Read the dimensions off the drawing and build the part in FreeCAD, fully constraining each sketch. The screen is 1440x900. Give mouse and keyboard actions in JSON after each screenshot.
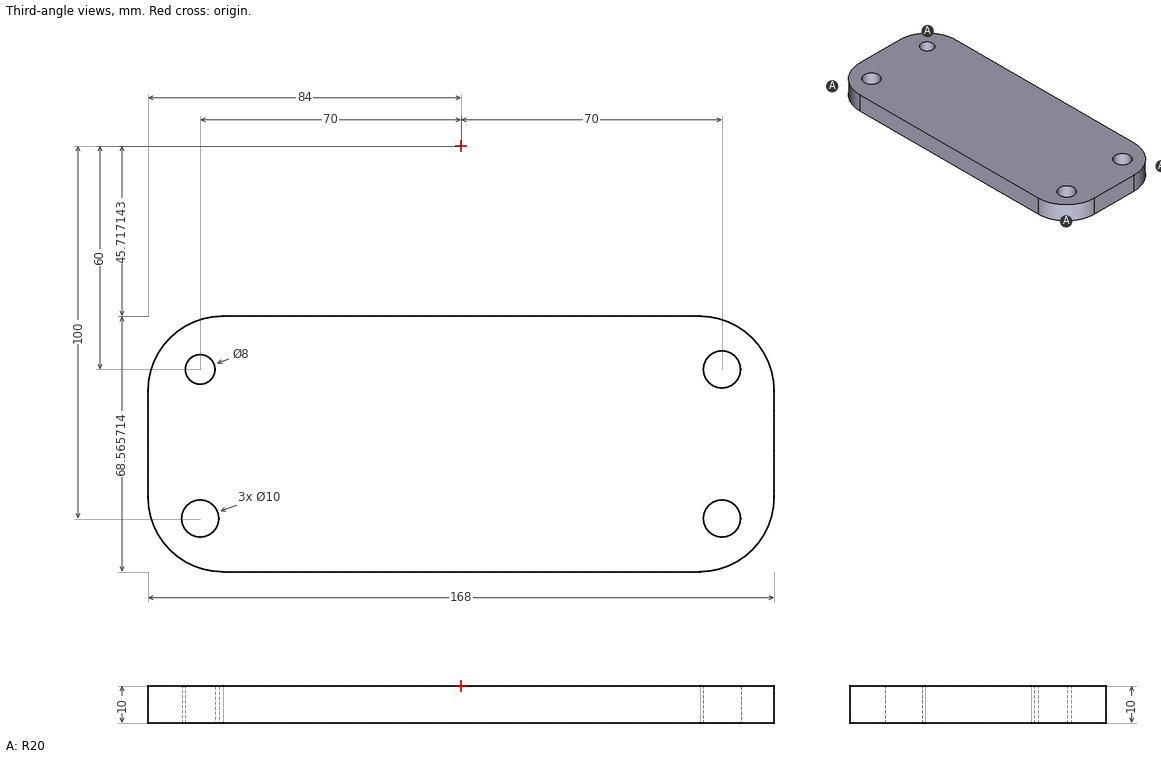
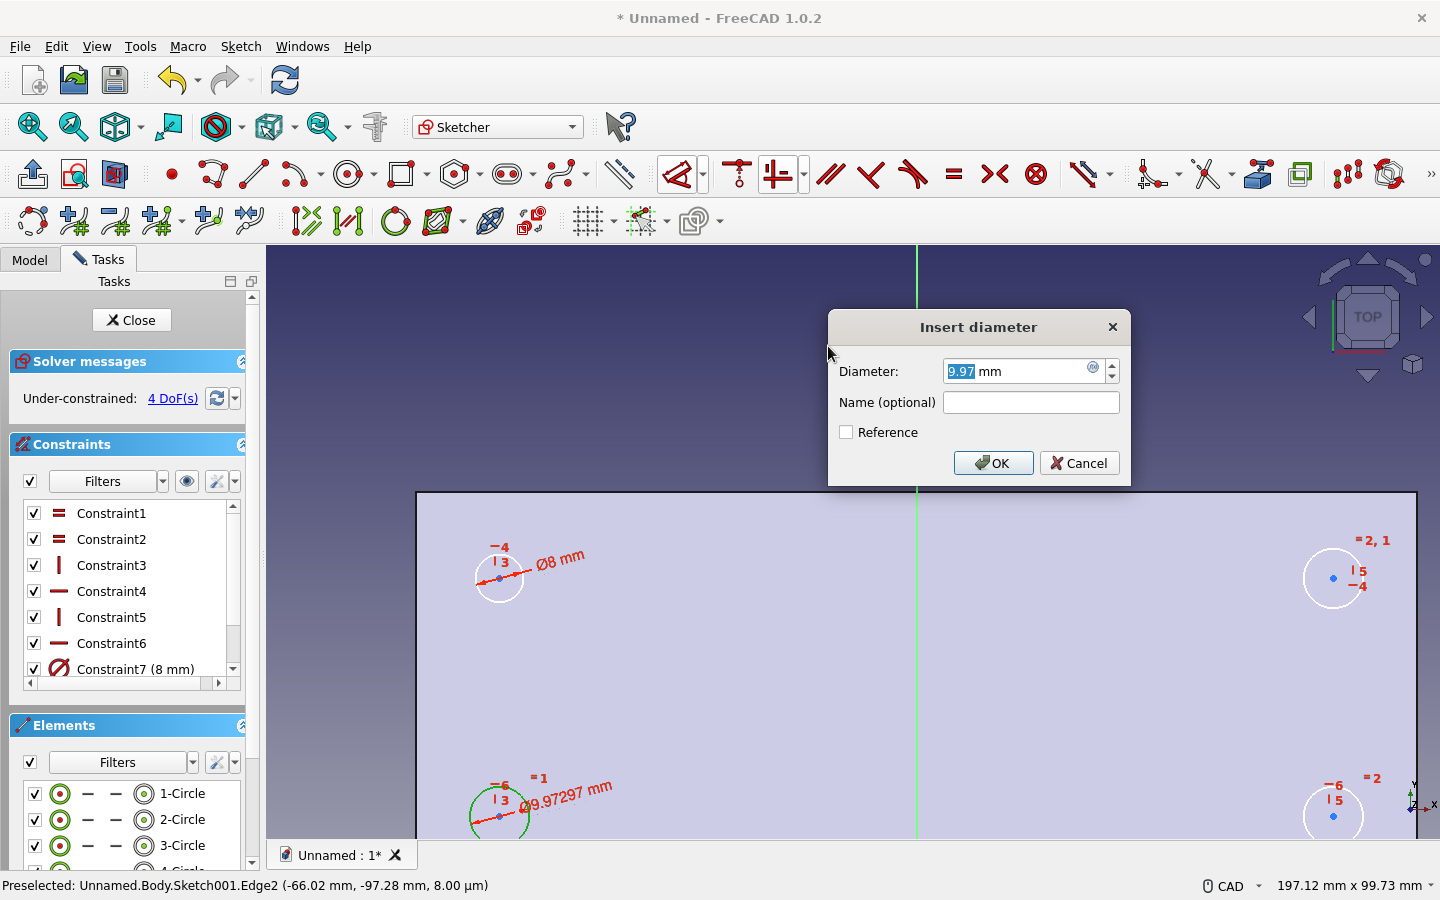
{"action": "type", "text": "10"}
{"action": "key", "text": "Return"}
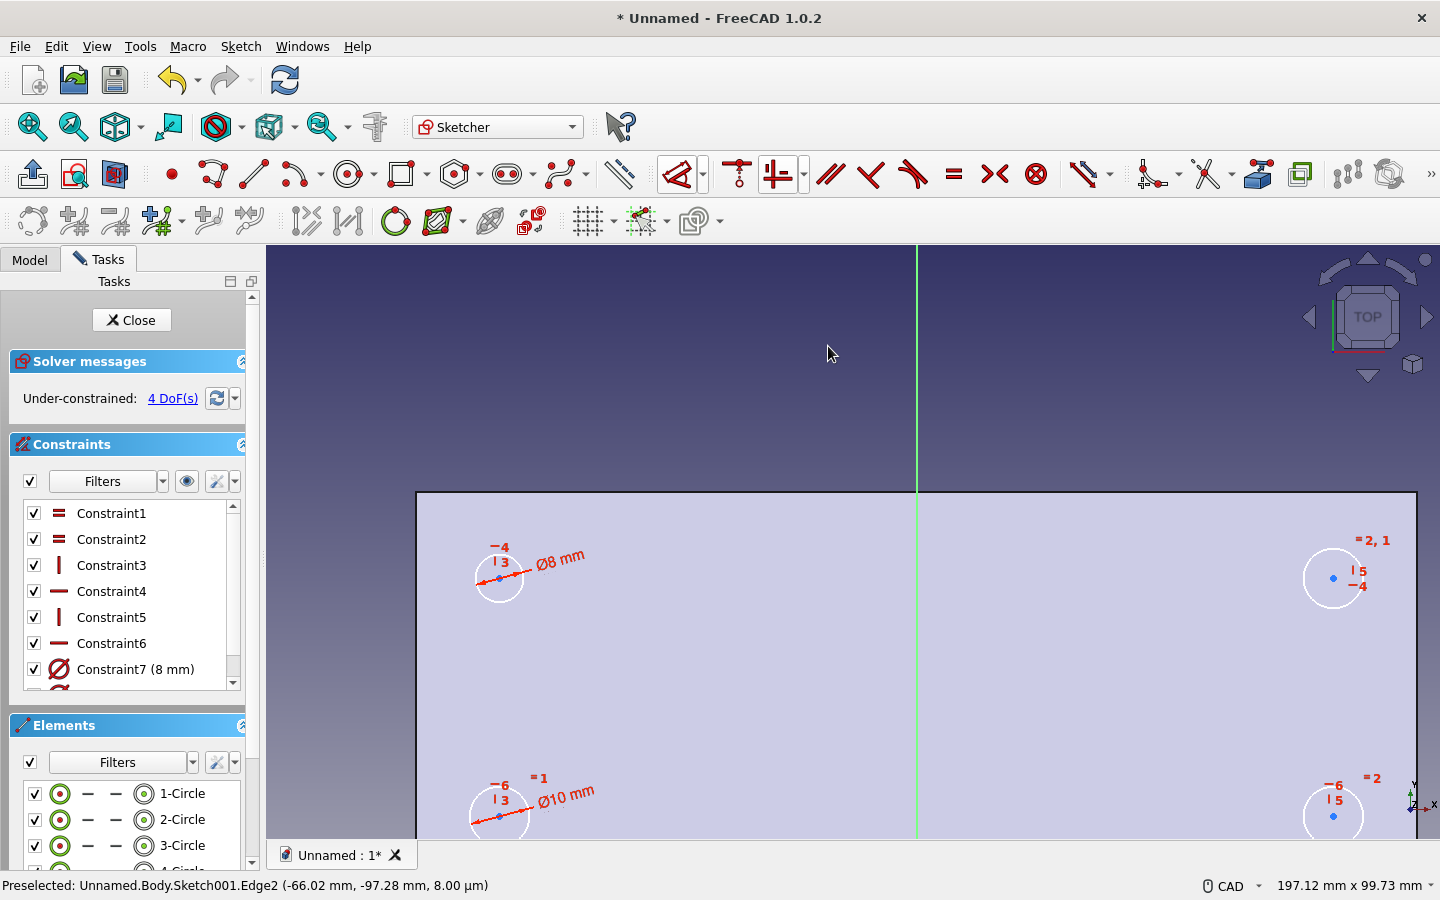
{"action": "left_click", "coordinate": [500, 578]}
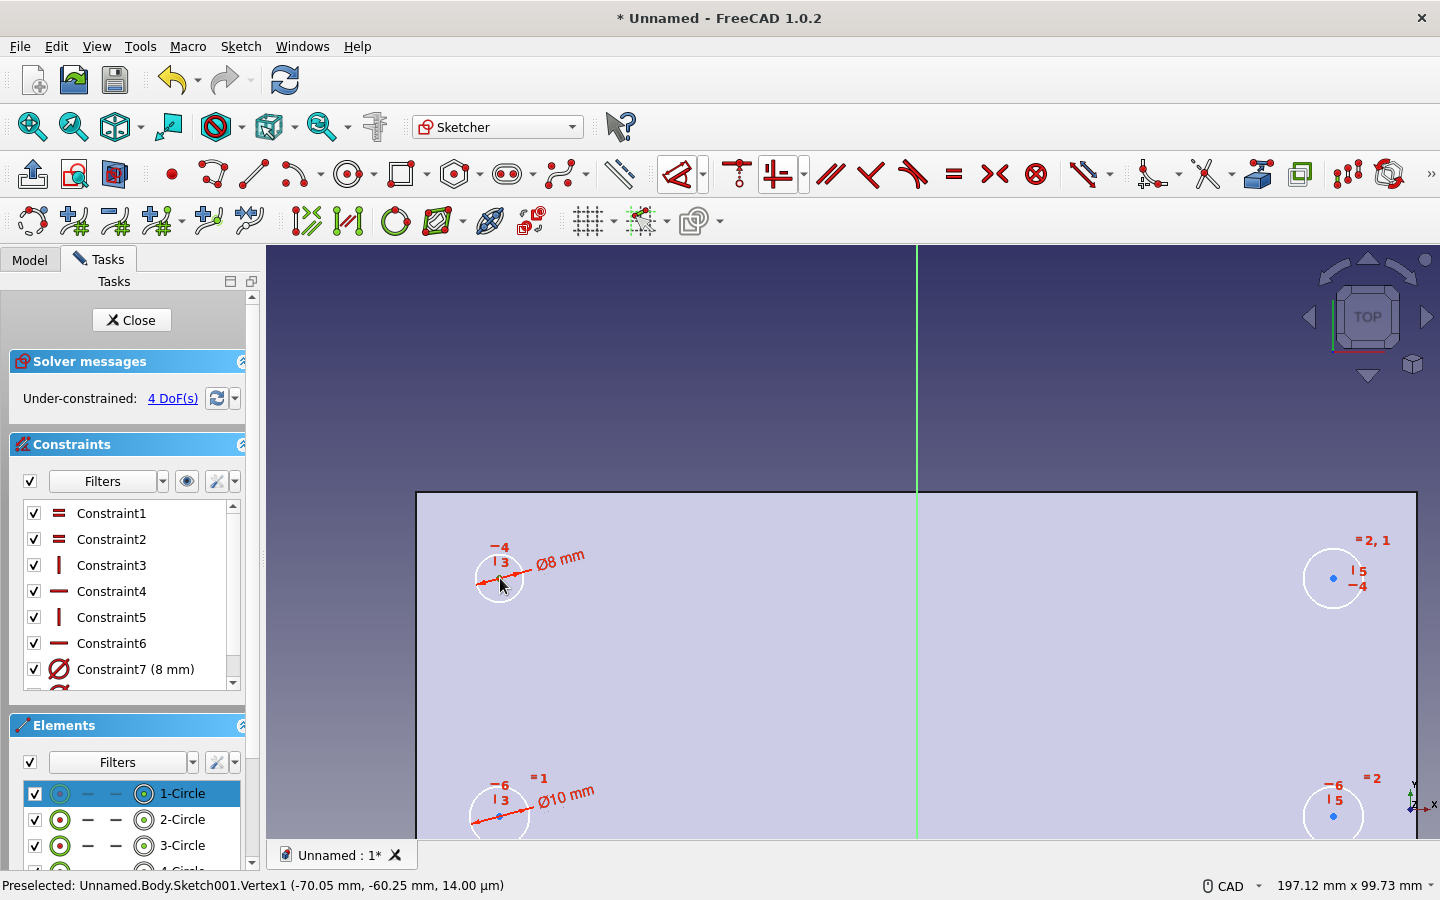
{"action": "left_click", "coordinate": [702, 174]}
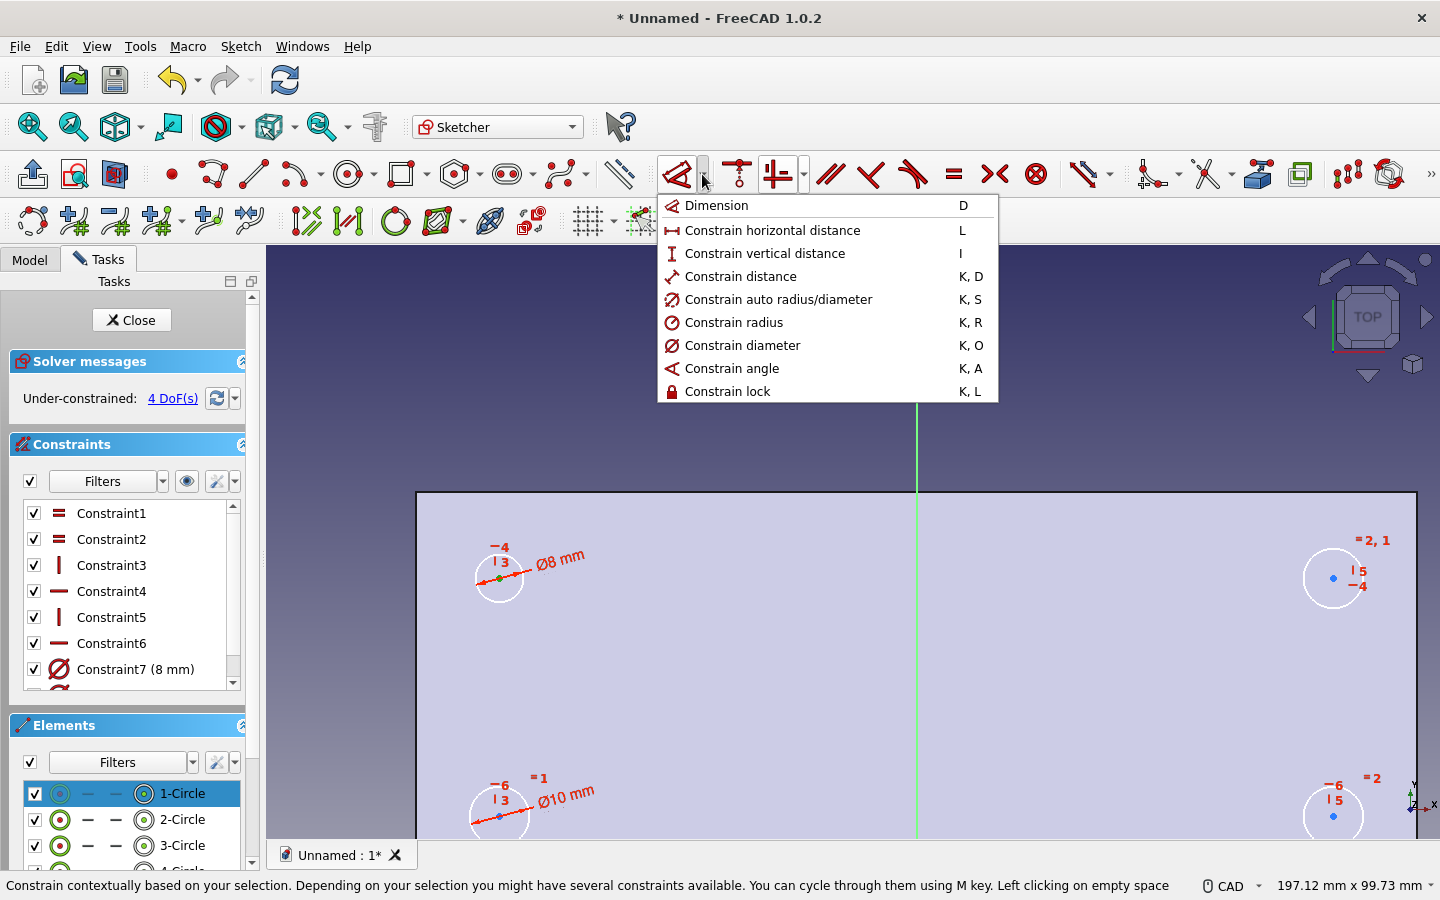
{"action": "left_click", "coordinate": [828, 230]}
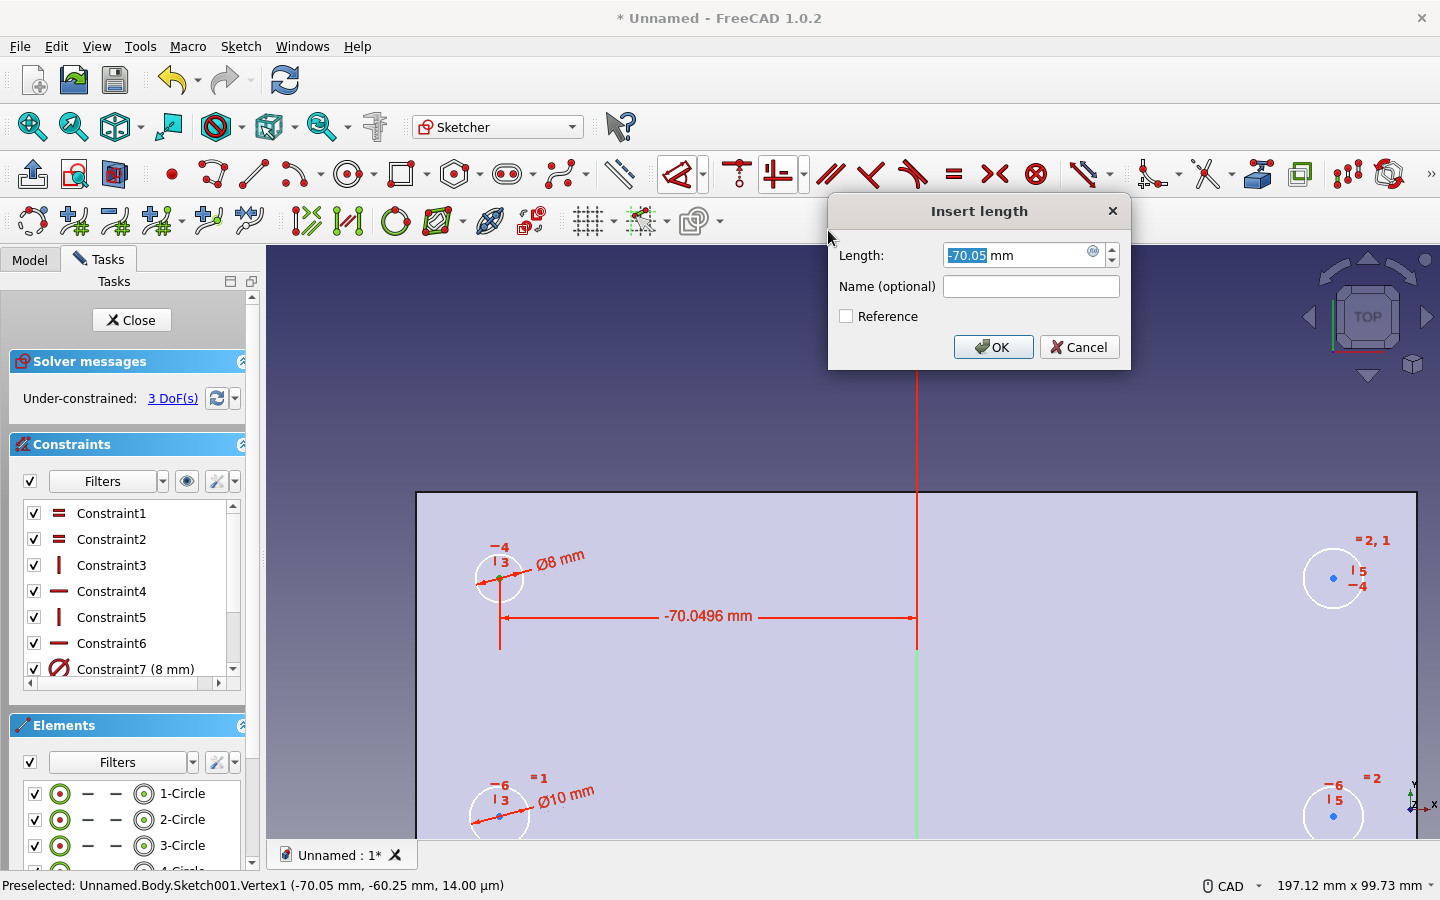
{"action": "type", "text": "-70"}
{"action": "key", "text": "Return"}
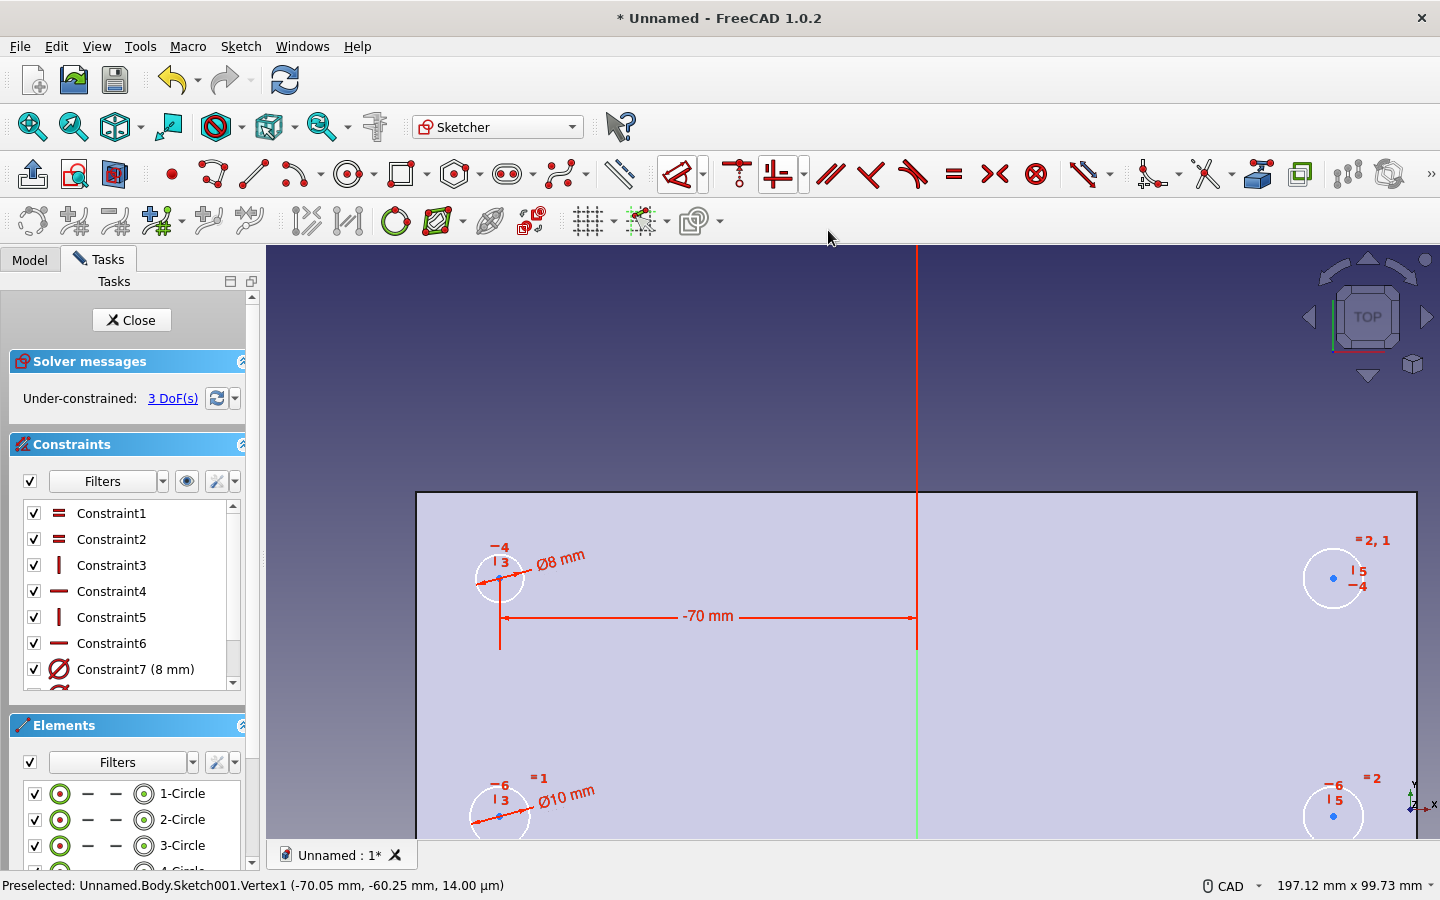
{"action": "left_click", "coordinate": [500, 578]}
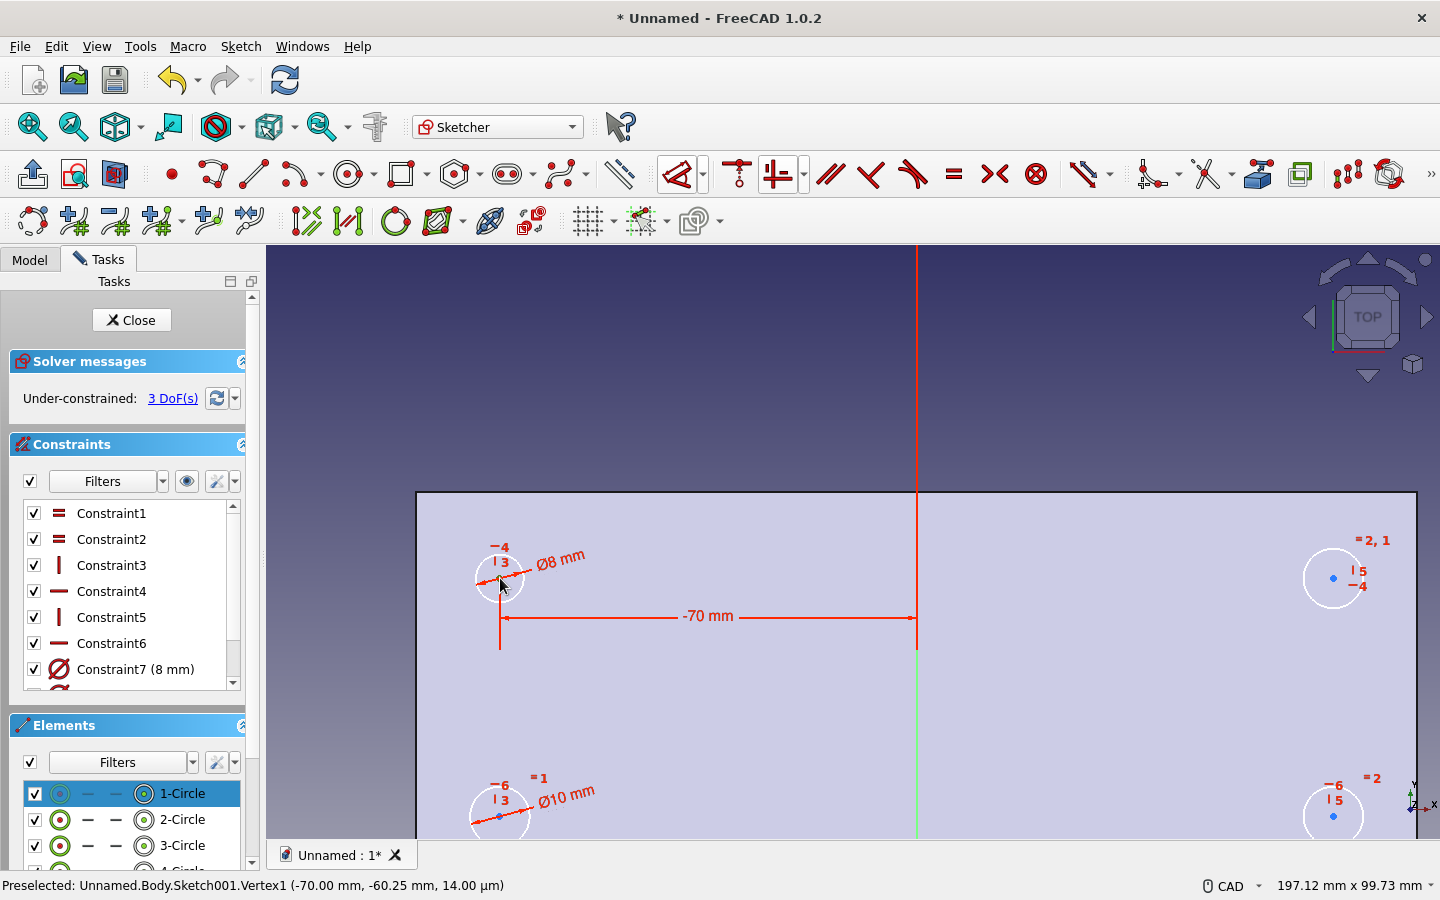
{"action": "key", "text": "i"}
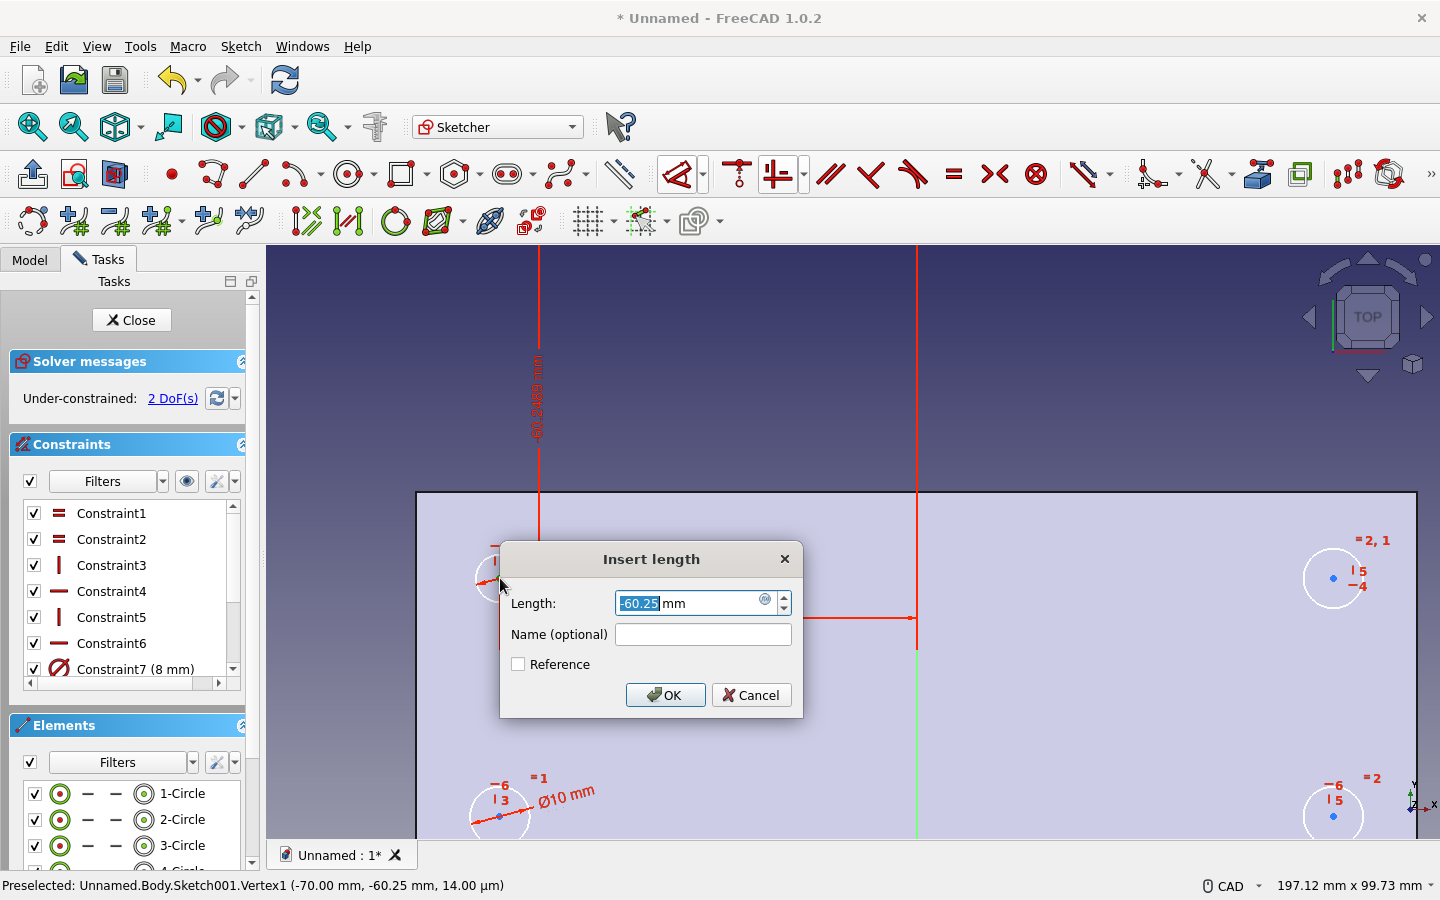
{"action": "type", "text": "-60"}
{"action": "key", "text": "Return"}